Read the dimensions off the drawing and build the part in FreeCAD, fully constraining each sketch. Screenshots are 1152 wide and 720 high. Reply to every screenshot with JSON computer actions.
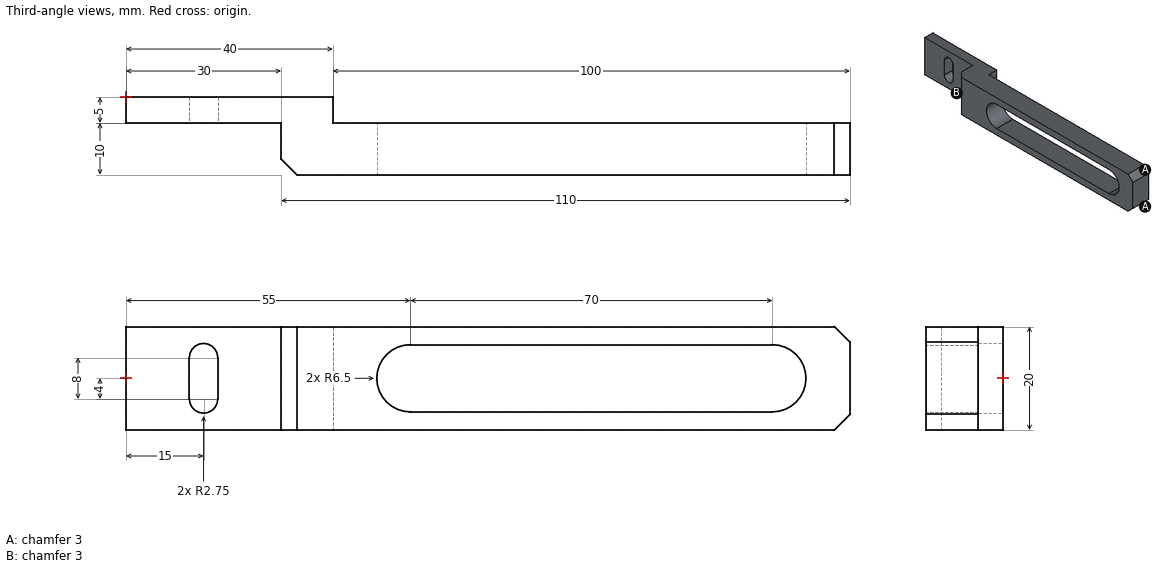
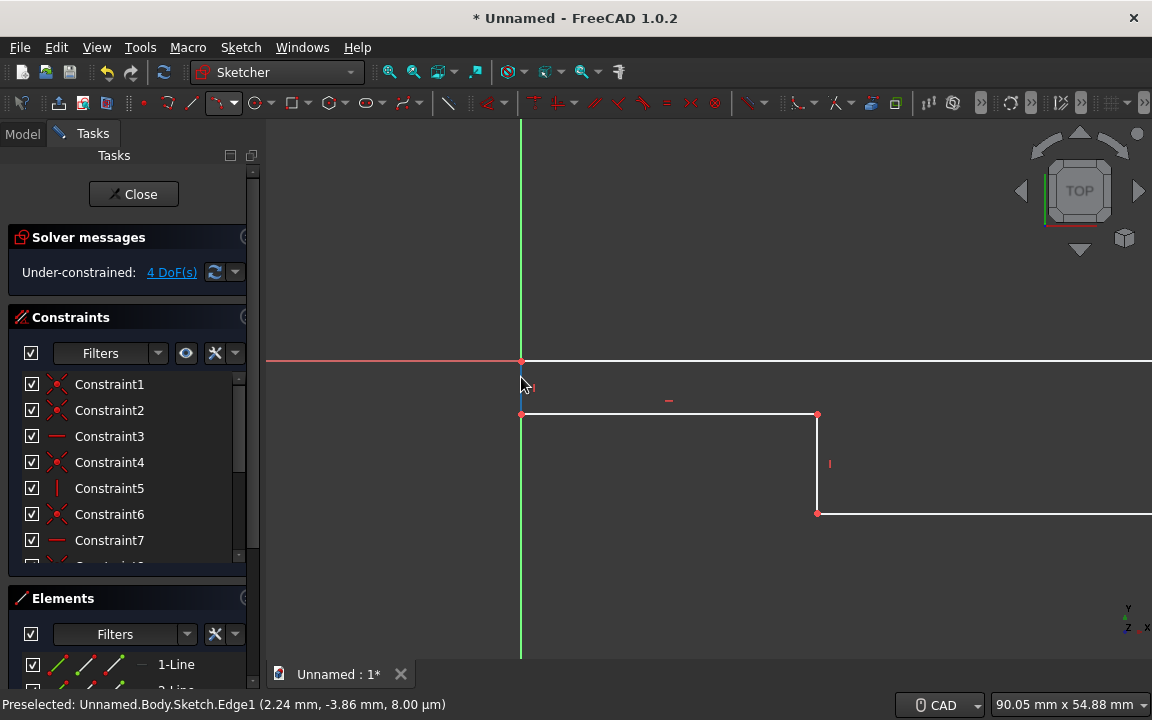
{"action": "left_click", "coordinate": [521, 377]}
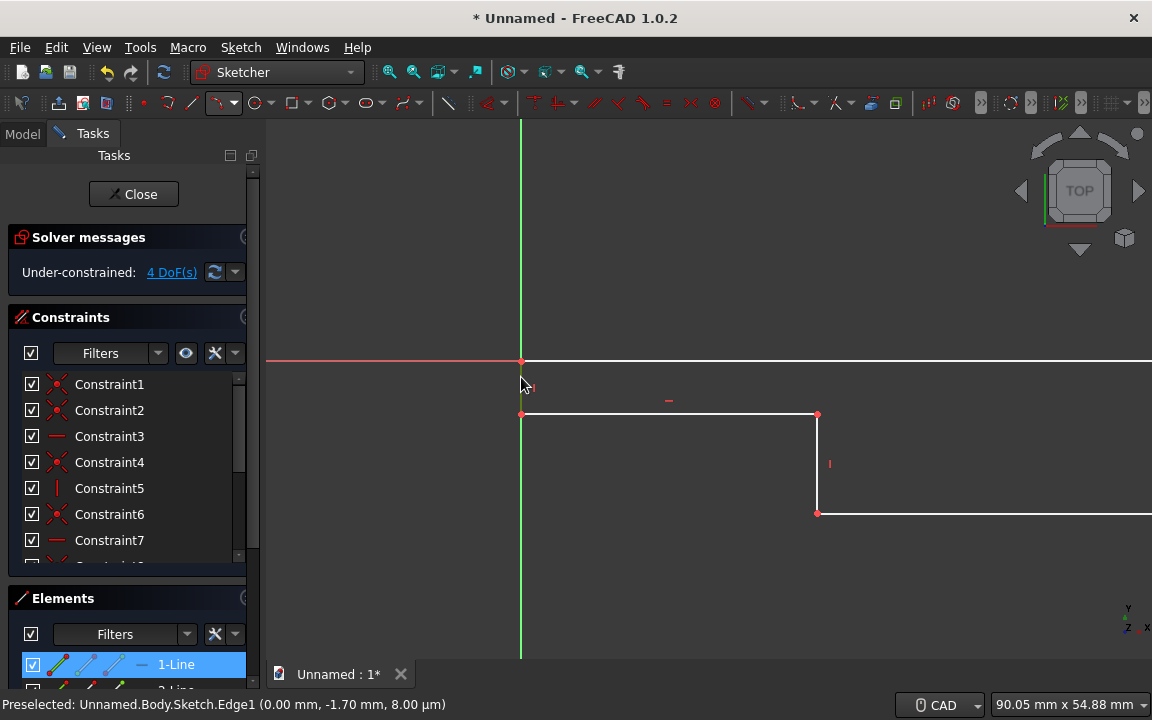
{"action": "key", "text": "i"}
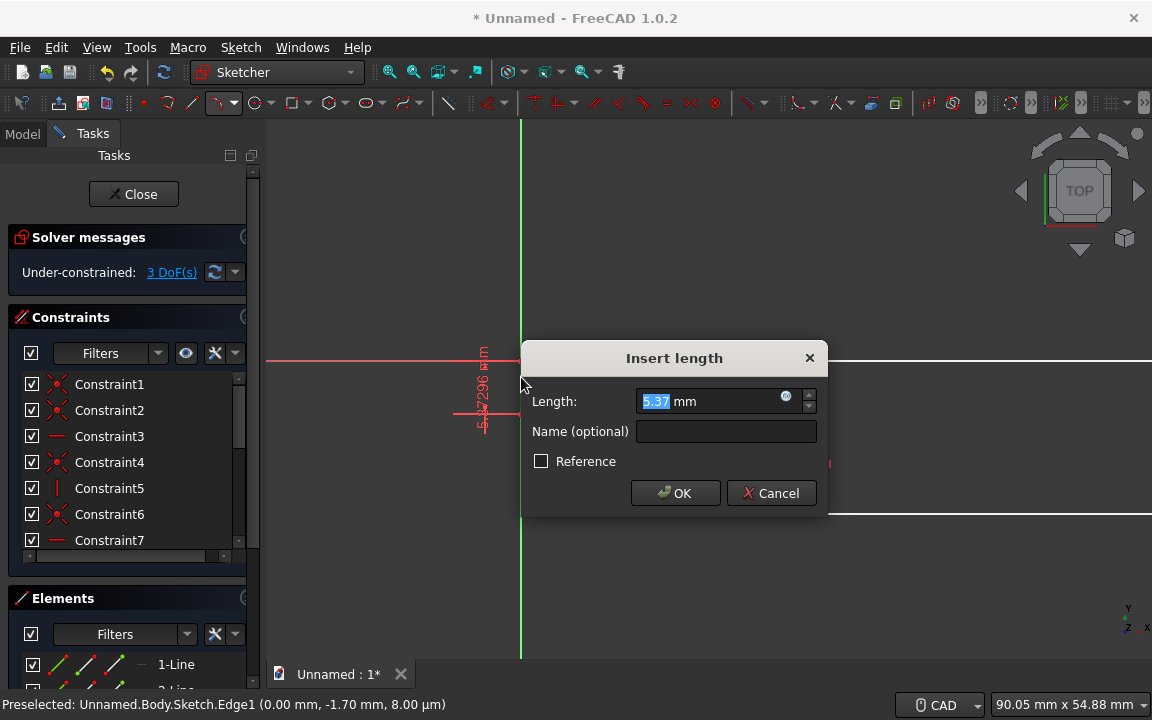
{"action": "type", "text": "5"}
{"action": "key", "text": "Return"}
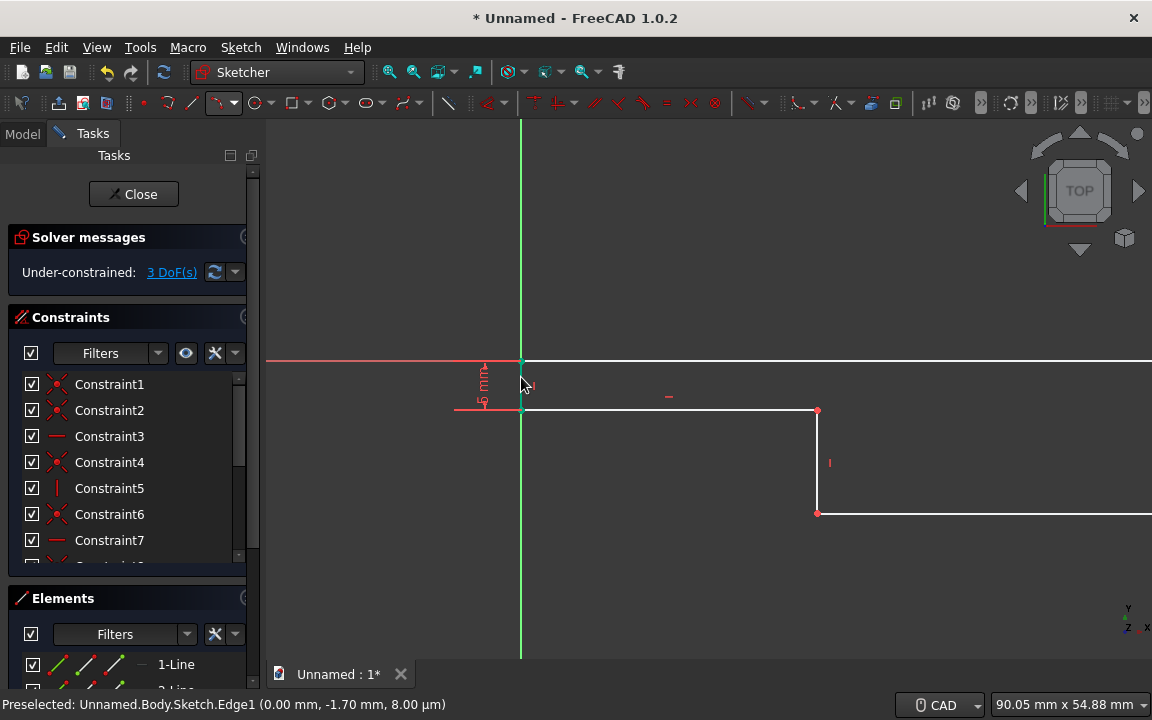
{"action": "left_click", "coordinate": [610, 410]}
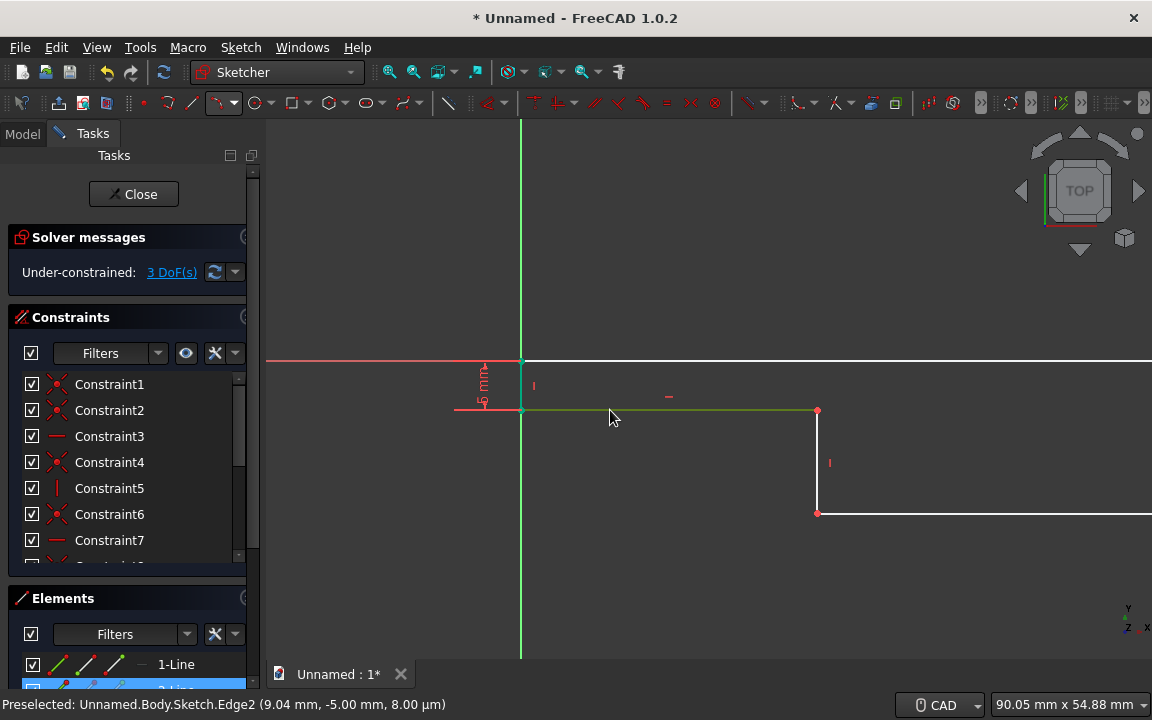
{"action": "left_click", "coordinate": [506, 104]}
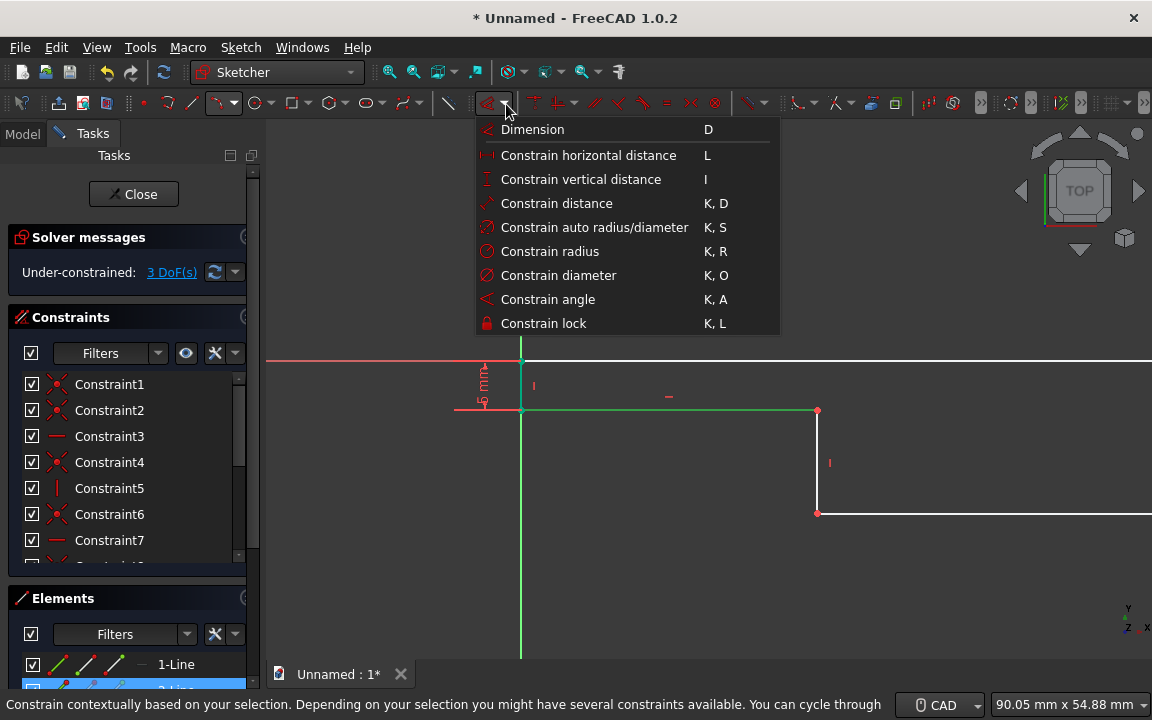
{"action": "left_click", "coordinate": [628, 155]}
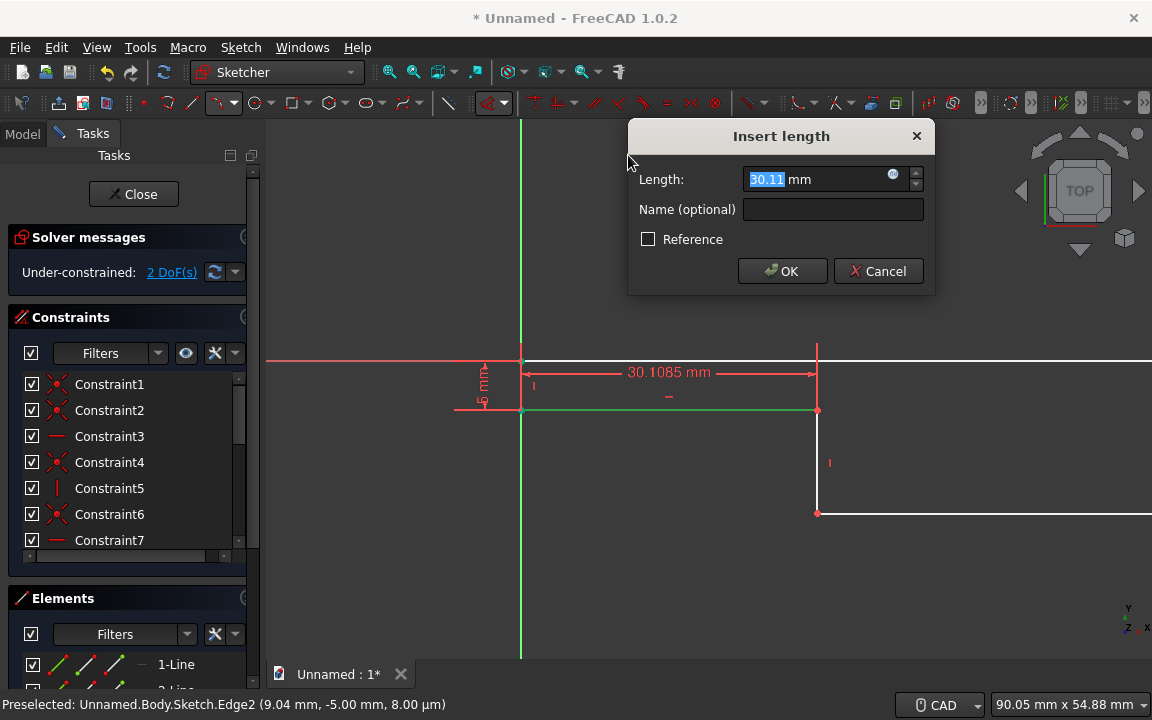
{"action": "type", "text": "30"}
{"action": "key", "text": "Return"}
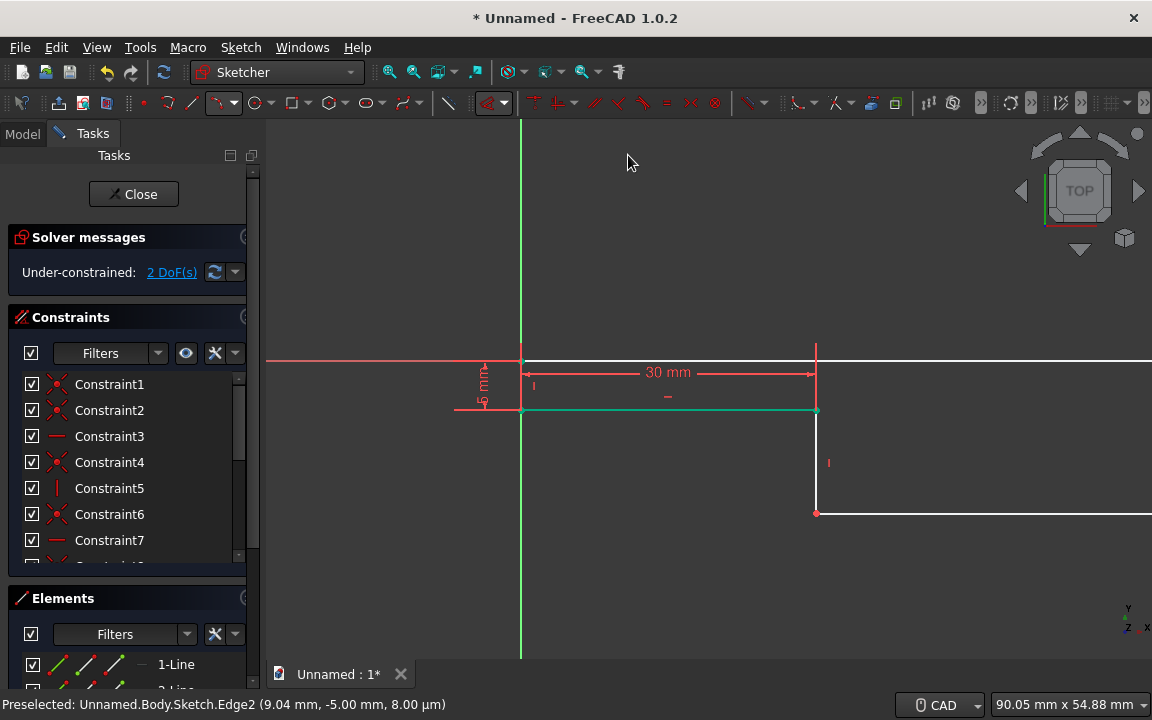
{"action": "left_click", "coordinate": [816, 441]}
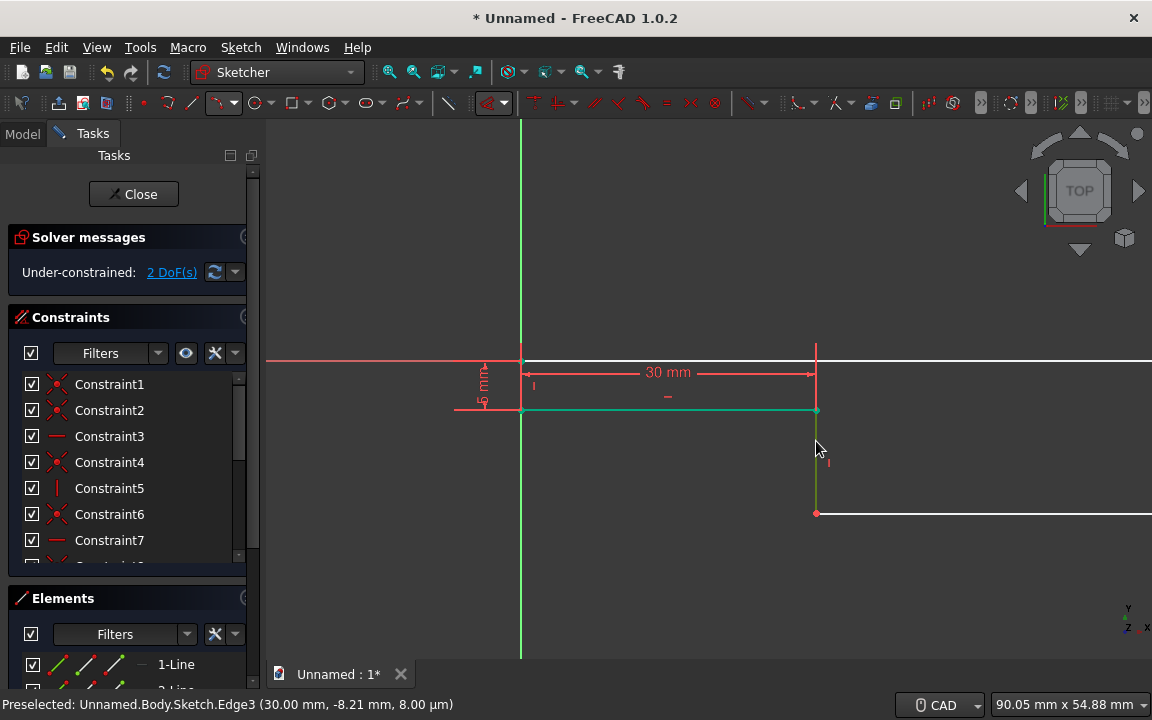
{"action": "key", "text": "i"}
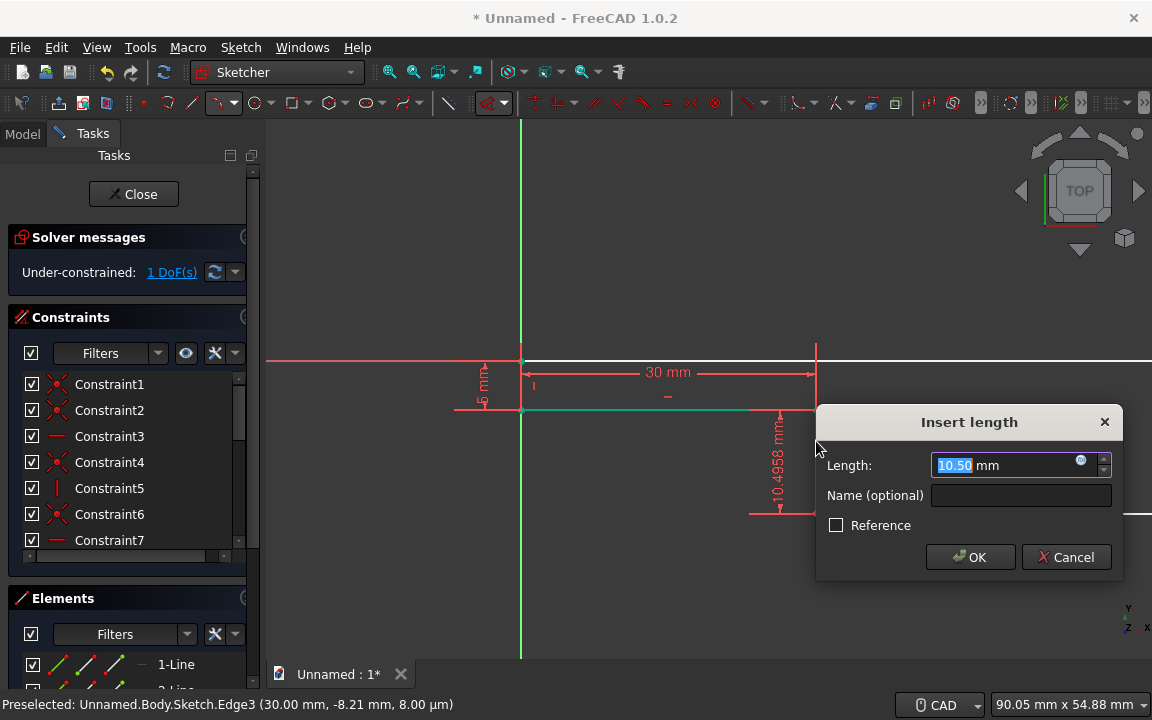
{"action": "type", "text": "10"}
{"action": "key", "text": "Return"}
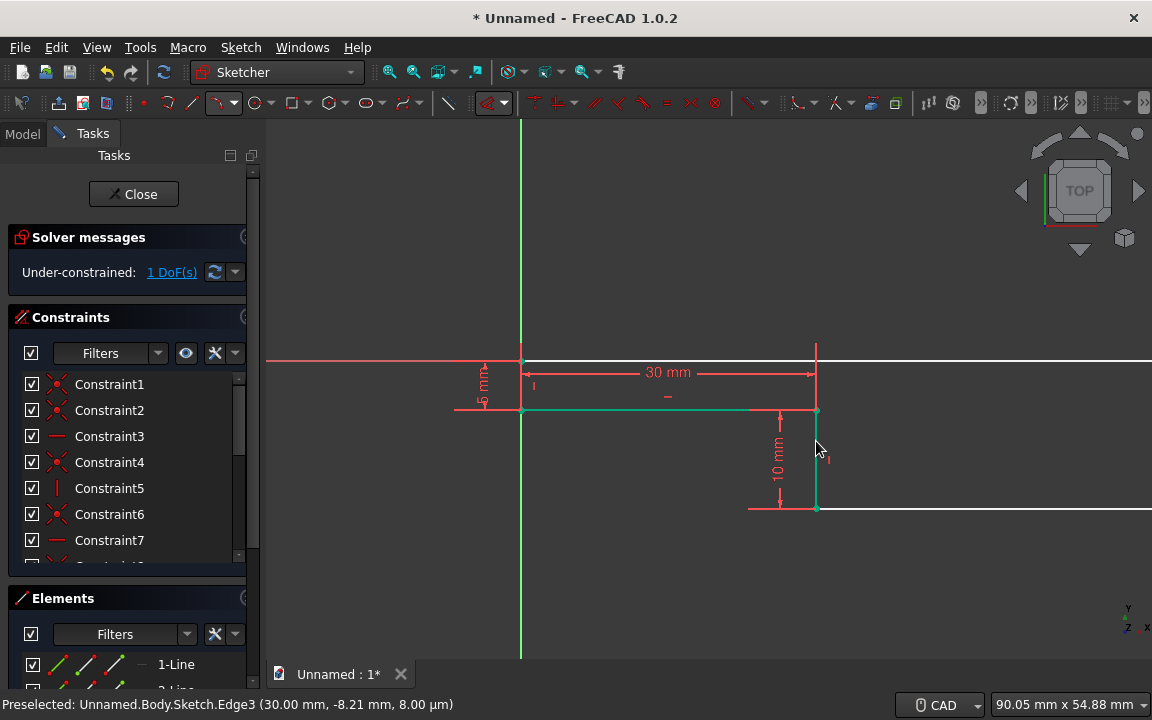
{"action": "scroll", "coordinate": [309, 362], "scroll_direction": "down", "scroll_amount": 5}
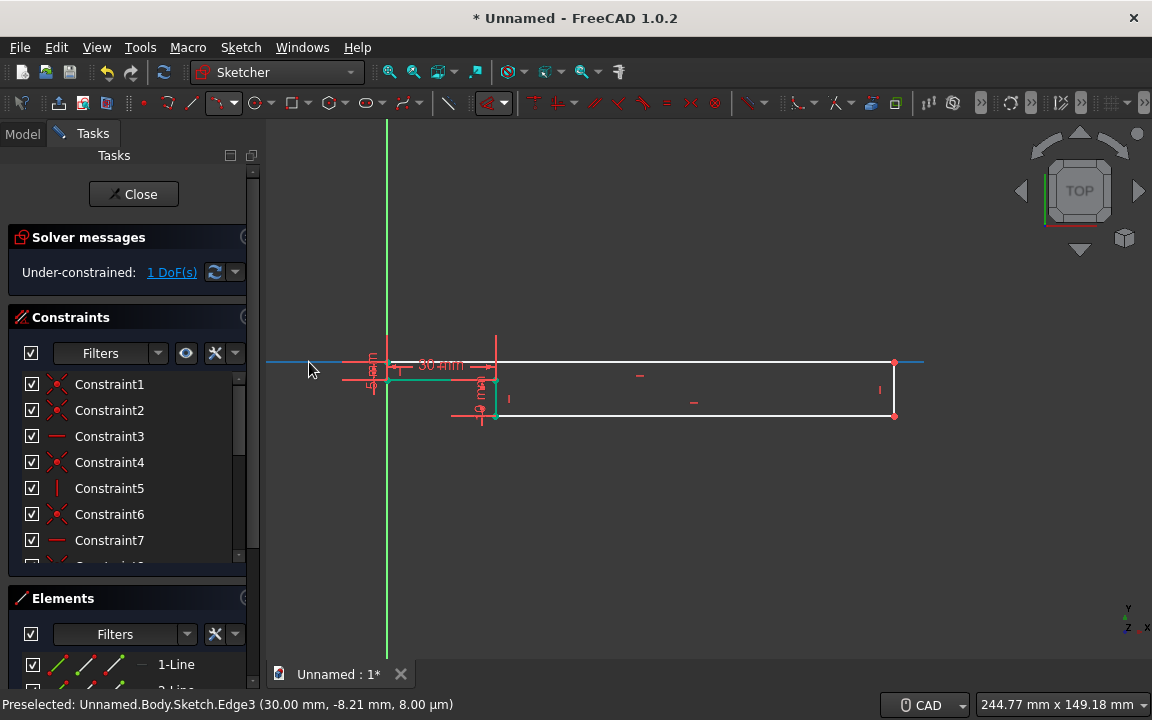
{"action": "left_click", "coordinate": [615, 416]}